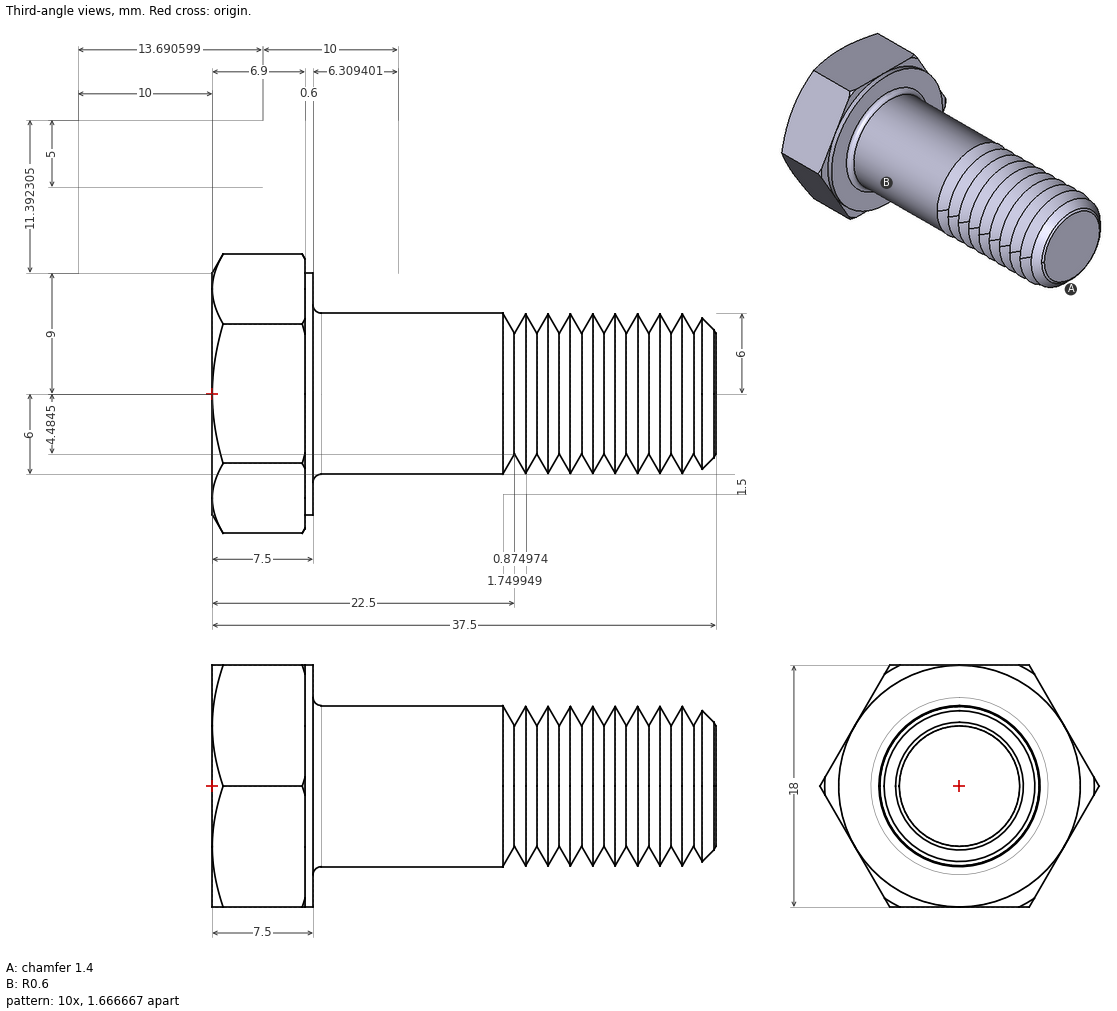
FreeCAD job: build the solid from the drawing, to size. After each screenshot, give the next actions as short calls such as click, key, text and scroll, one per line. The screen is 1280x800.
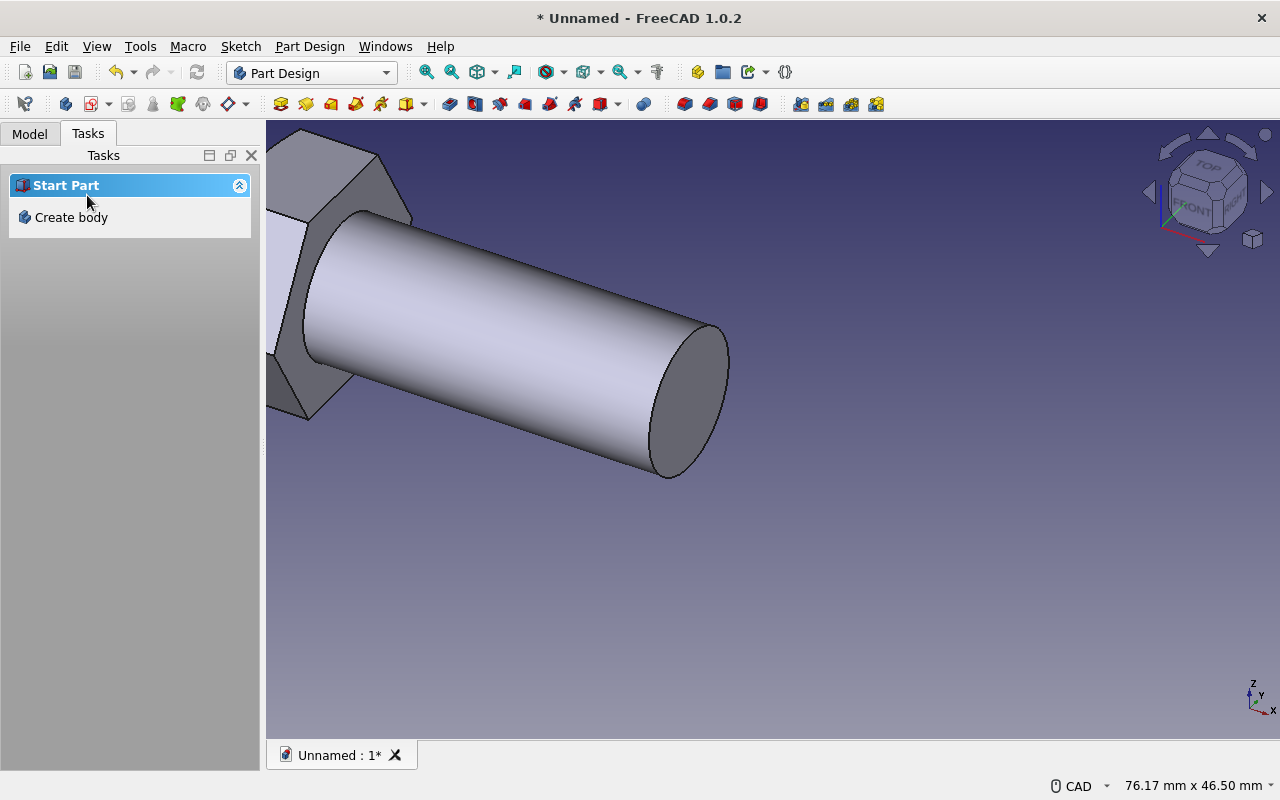
click(427, 72)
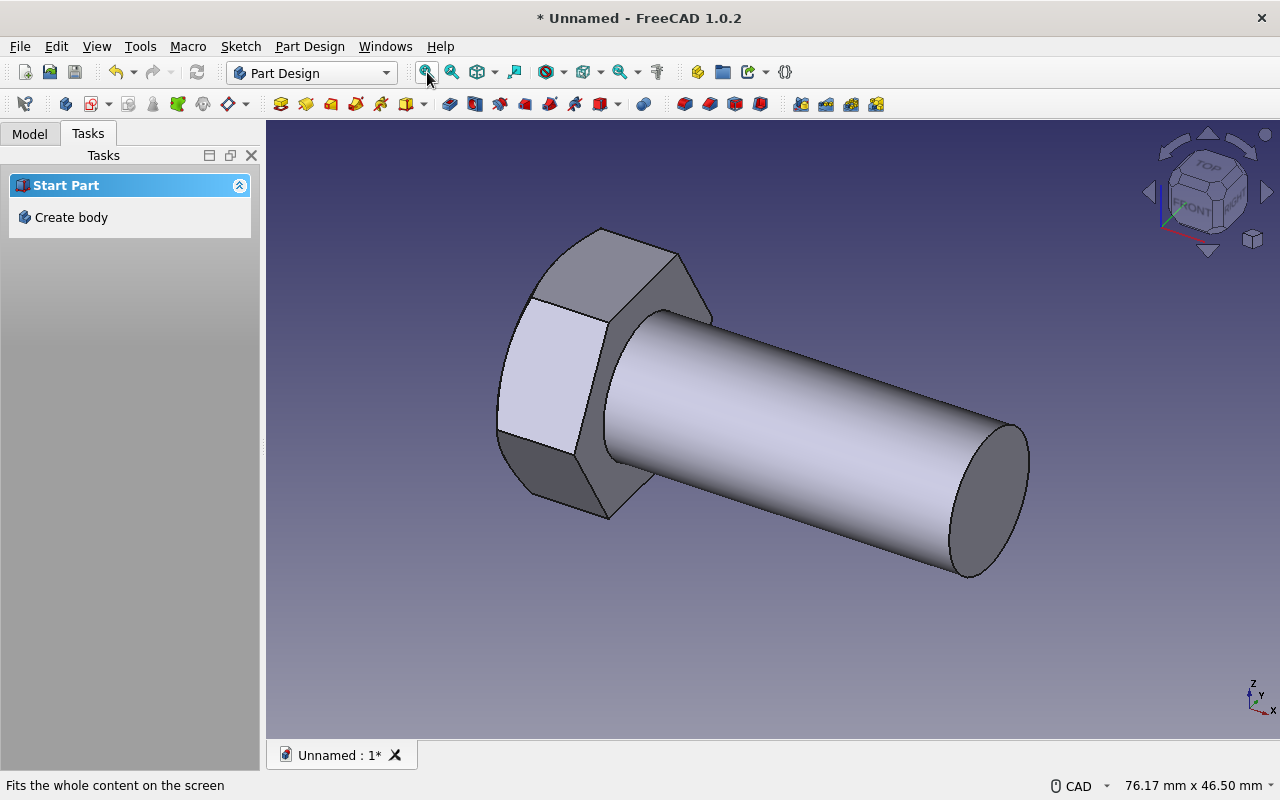
click(90, 104)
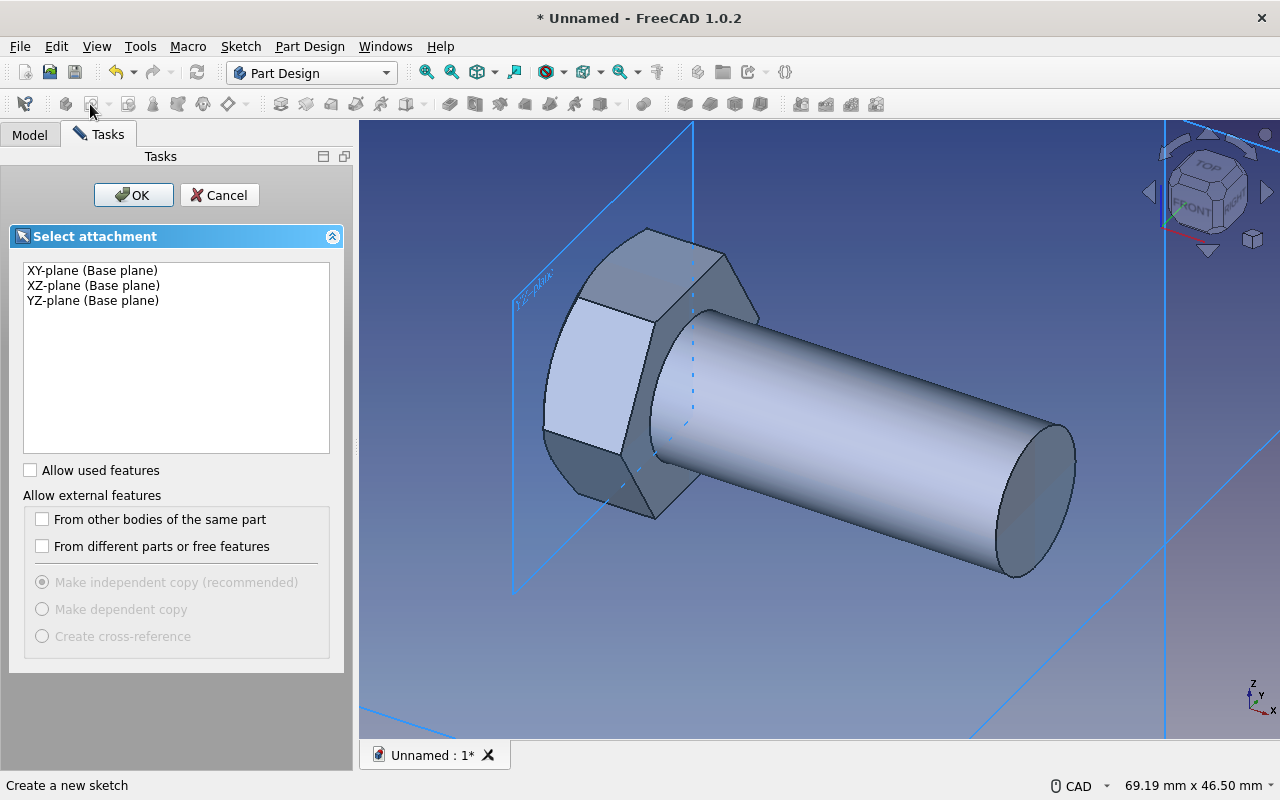
click(84, 270)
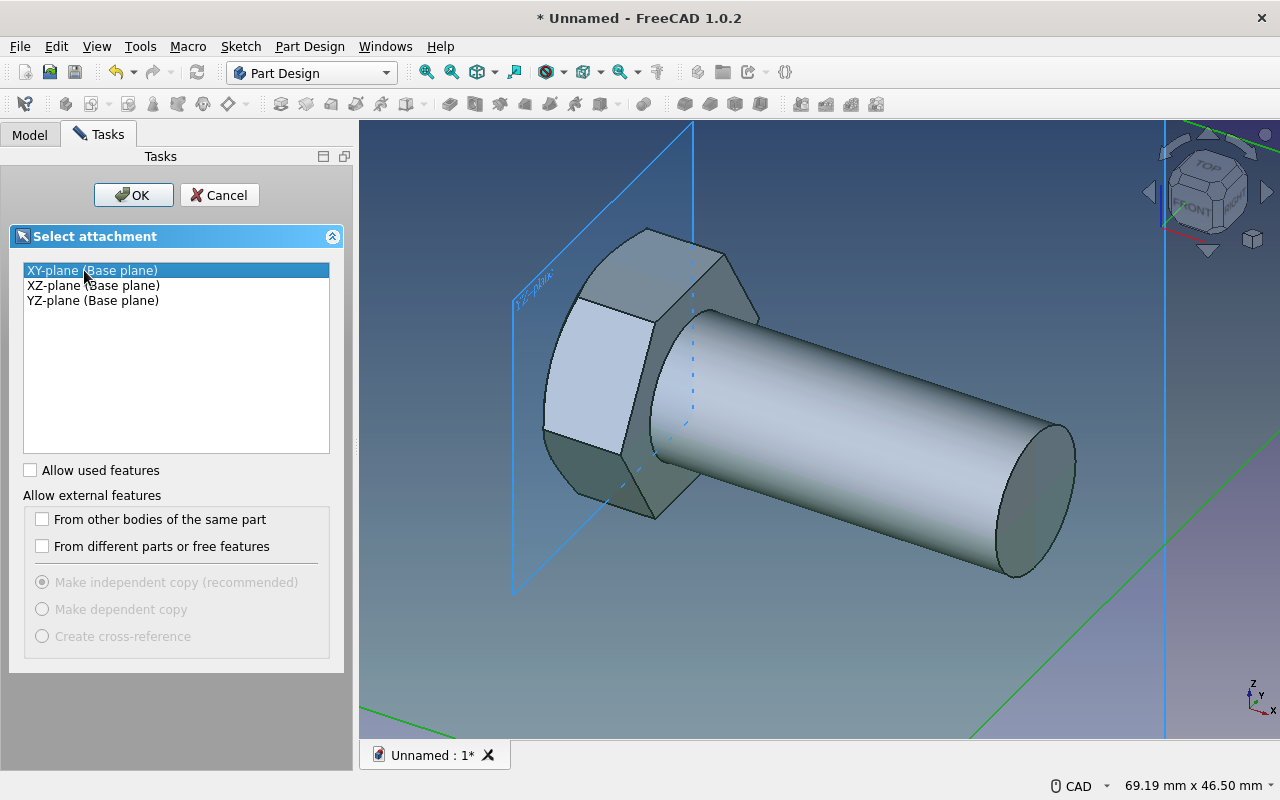
click(134, 195)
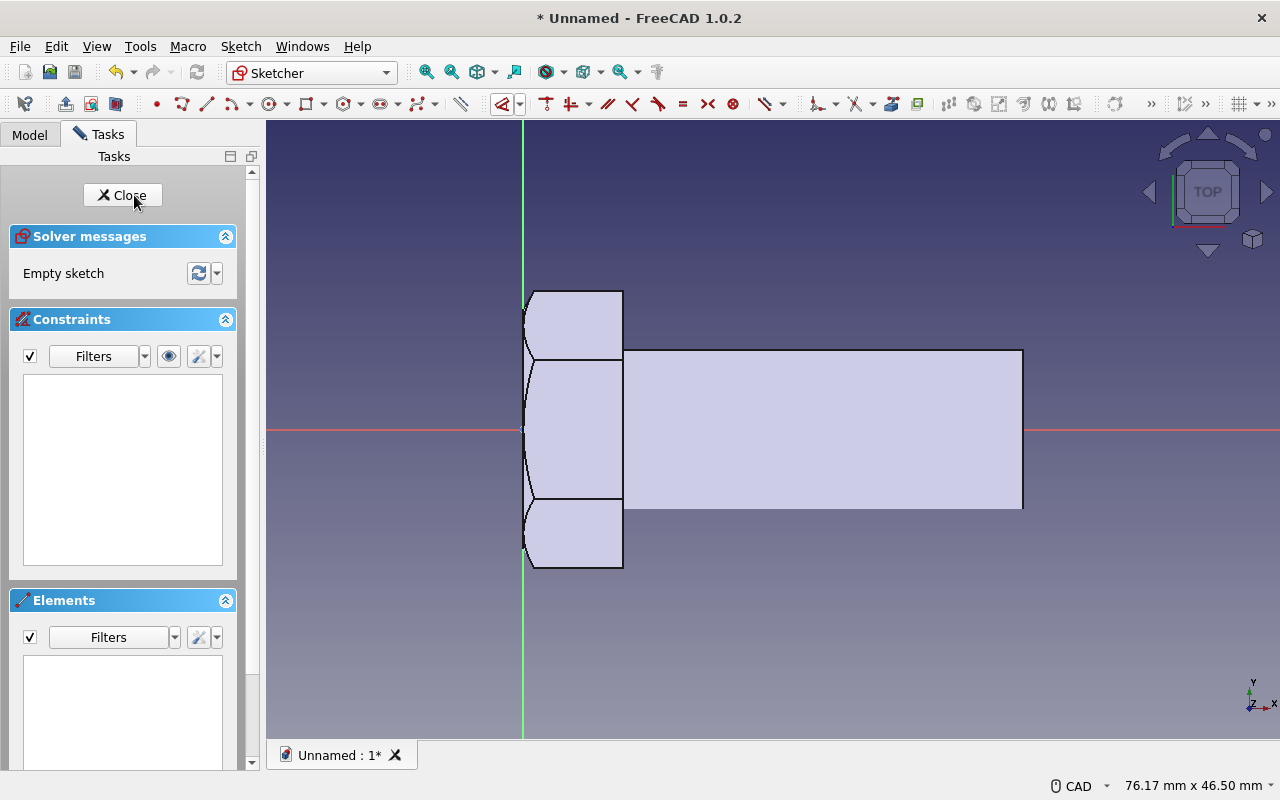
click(116, 104)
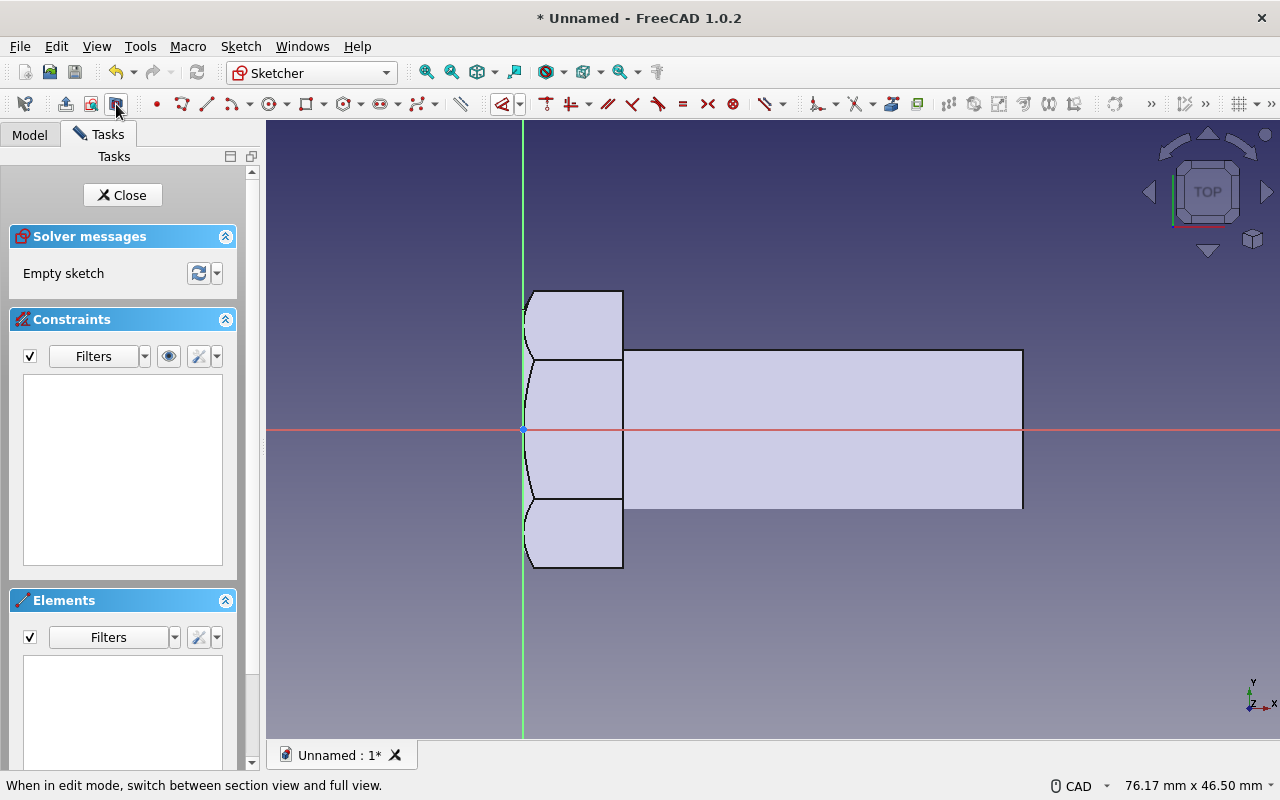
scroll(1107, 711, down, 1)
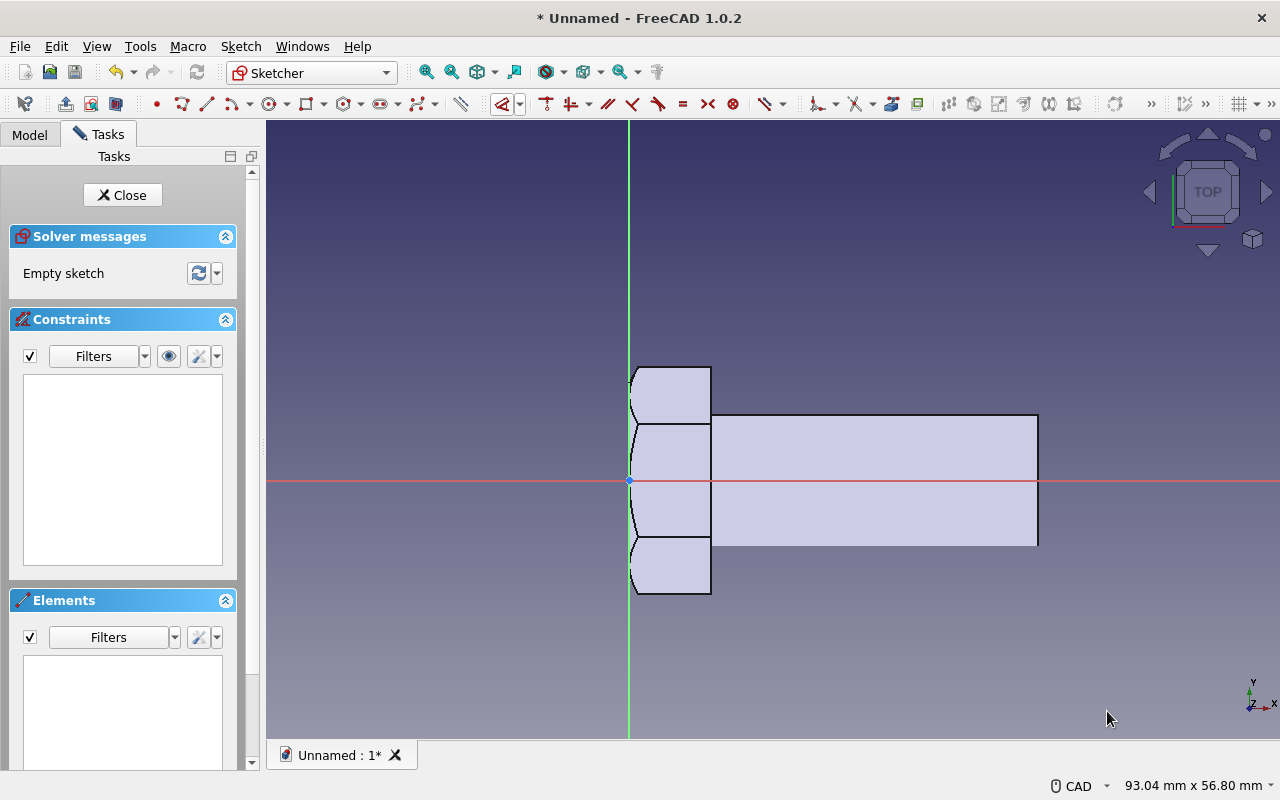
scroll(705, 297, up, 3)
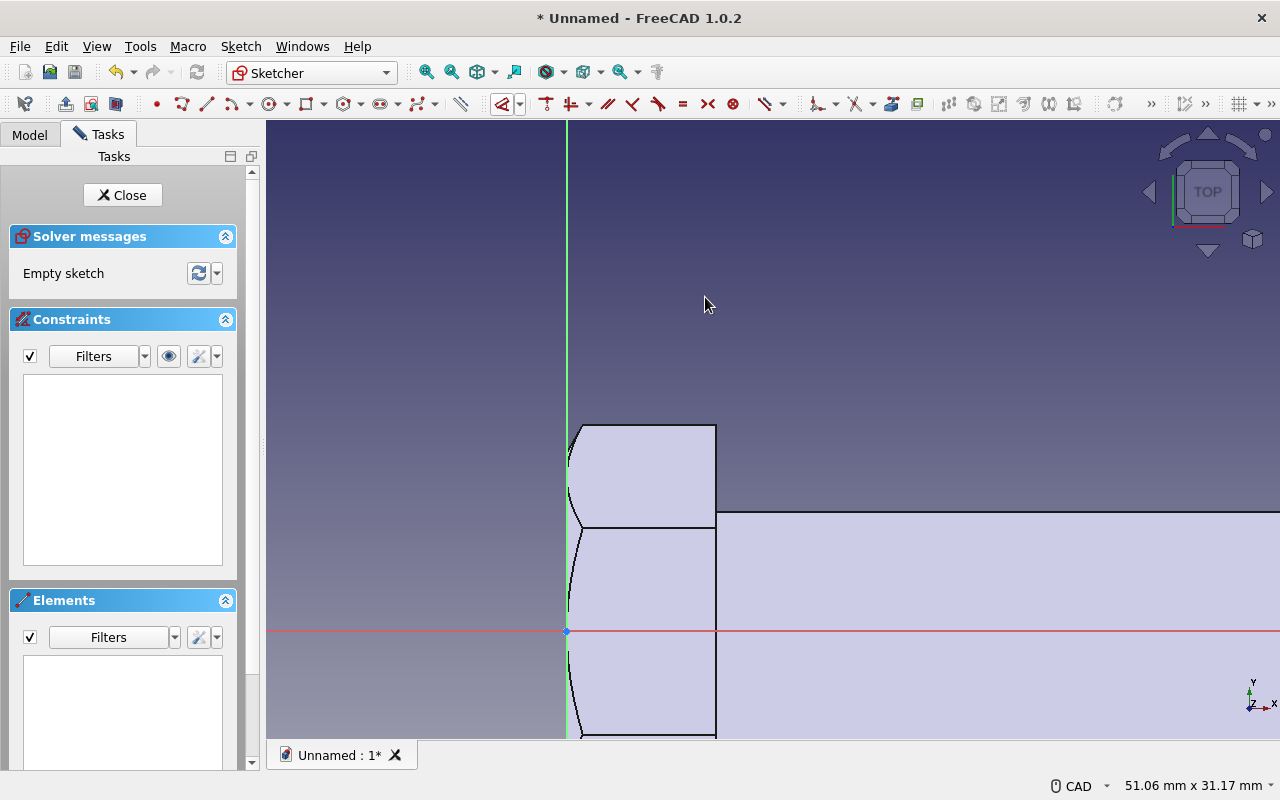
click(182, 104)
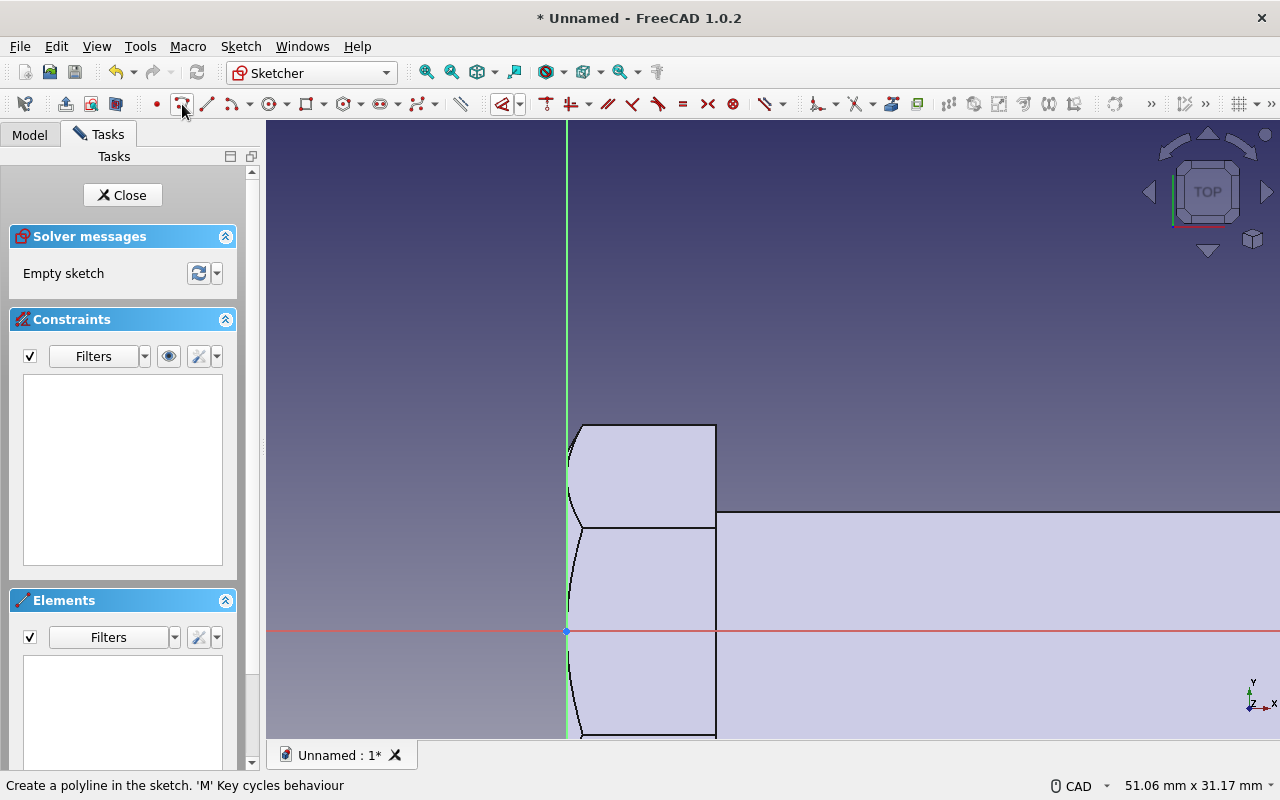
click(716, 453)
click(841, 453)
click(841, 227)
click(642, 227)
click(642, 326)
click(716, 454)
key(Escape)
key(Escape)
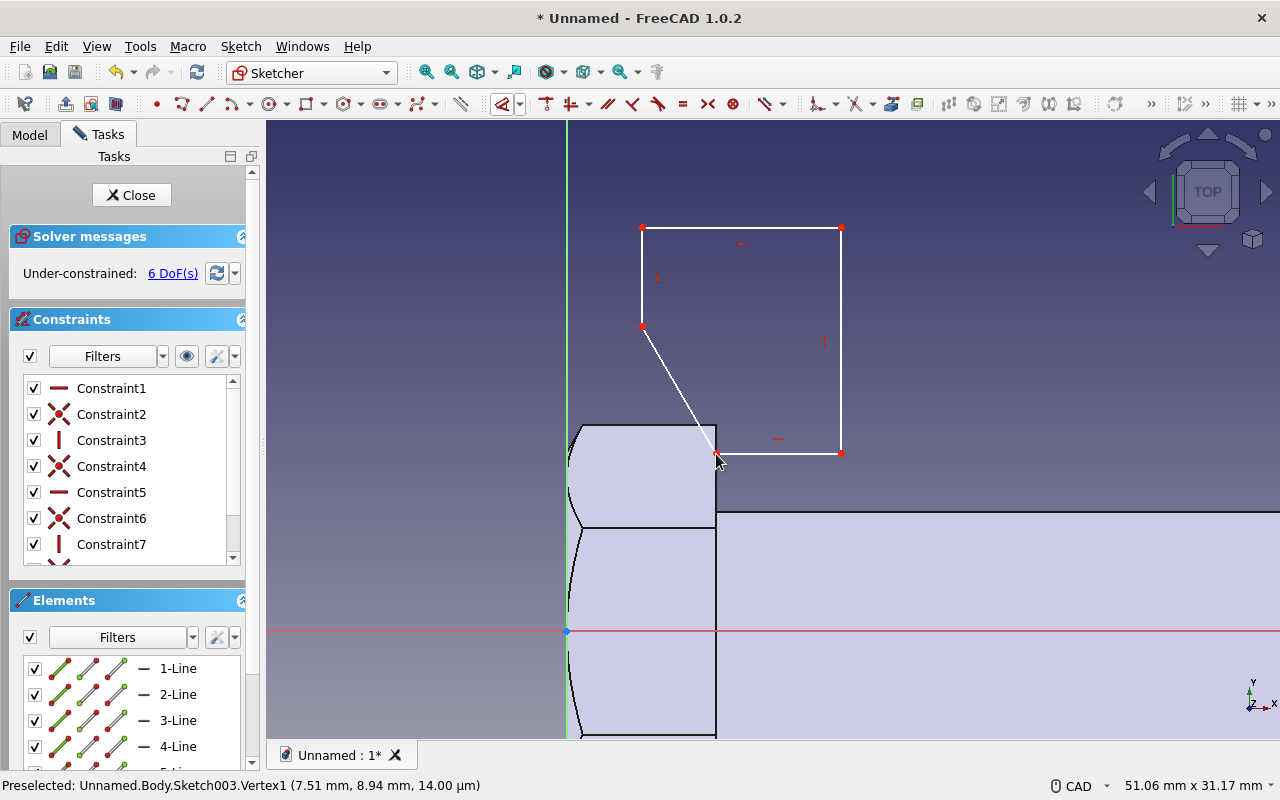
click(642, 258)